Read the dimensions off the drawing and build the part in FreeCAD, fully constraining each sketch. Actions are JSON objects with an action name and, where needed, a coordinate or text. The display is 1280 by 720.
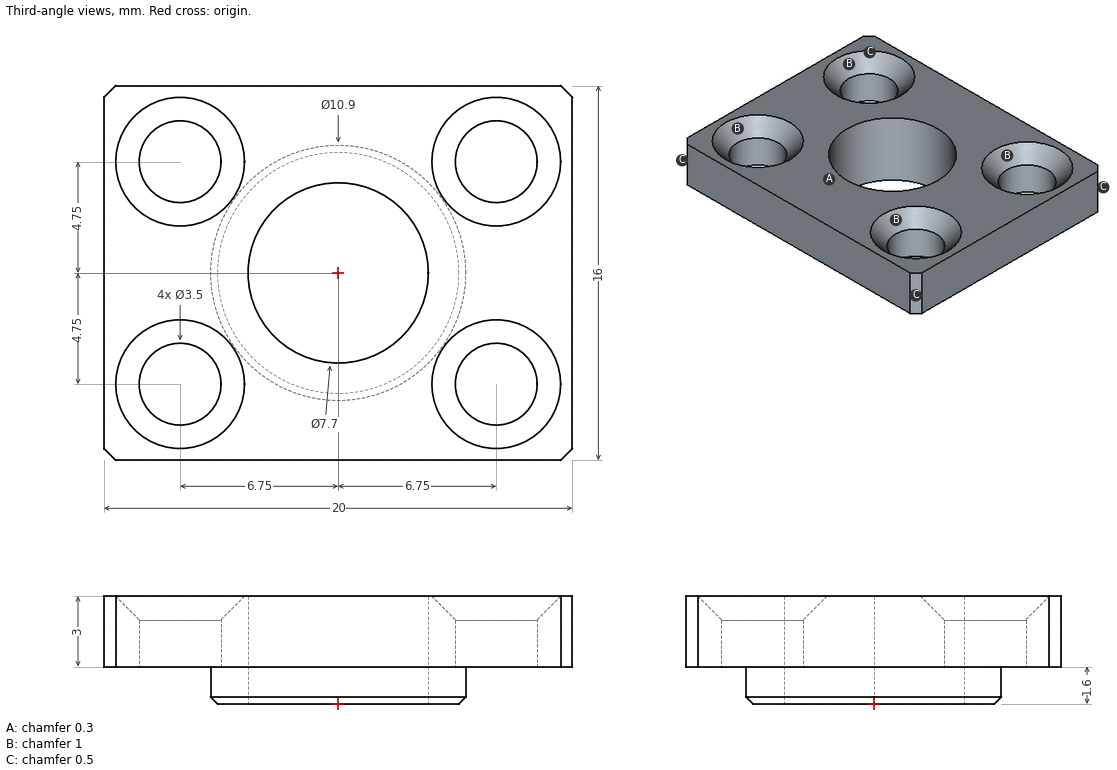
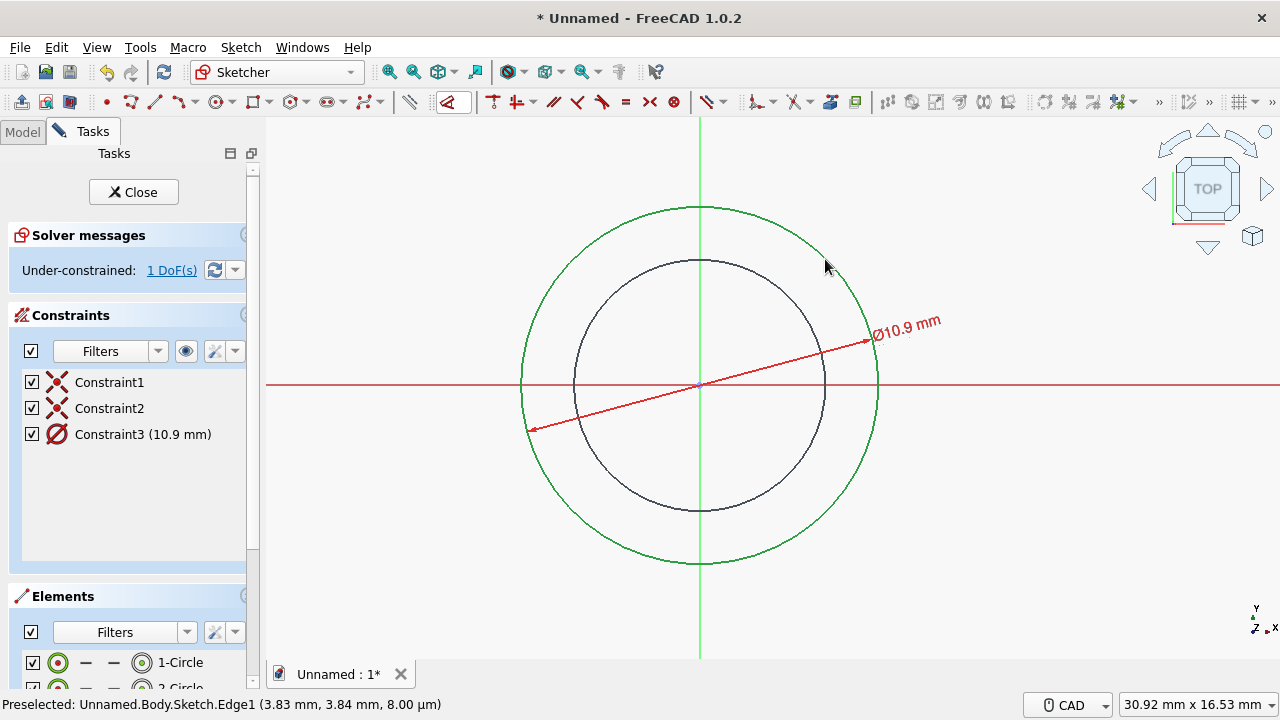
{"action": "left_click", "coordinate": [788, 296]}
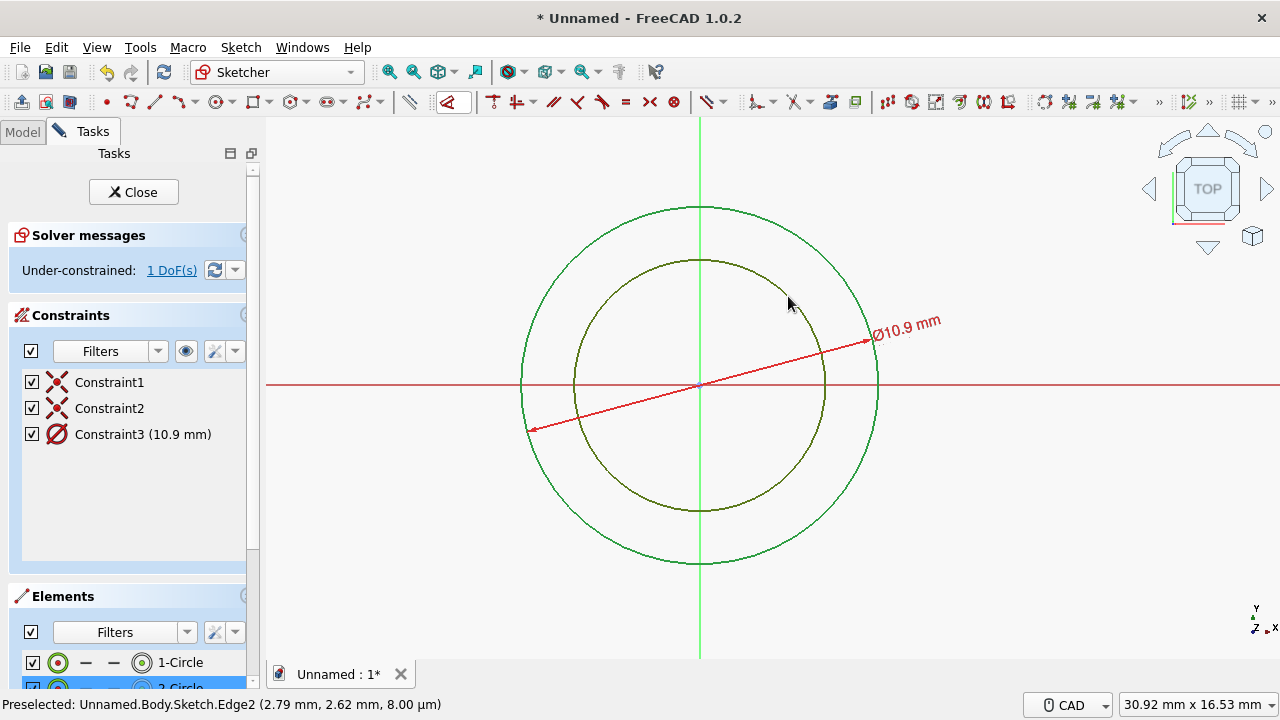
{"action": "key", "text": "k o"}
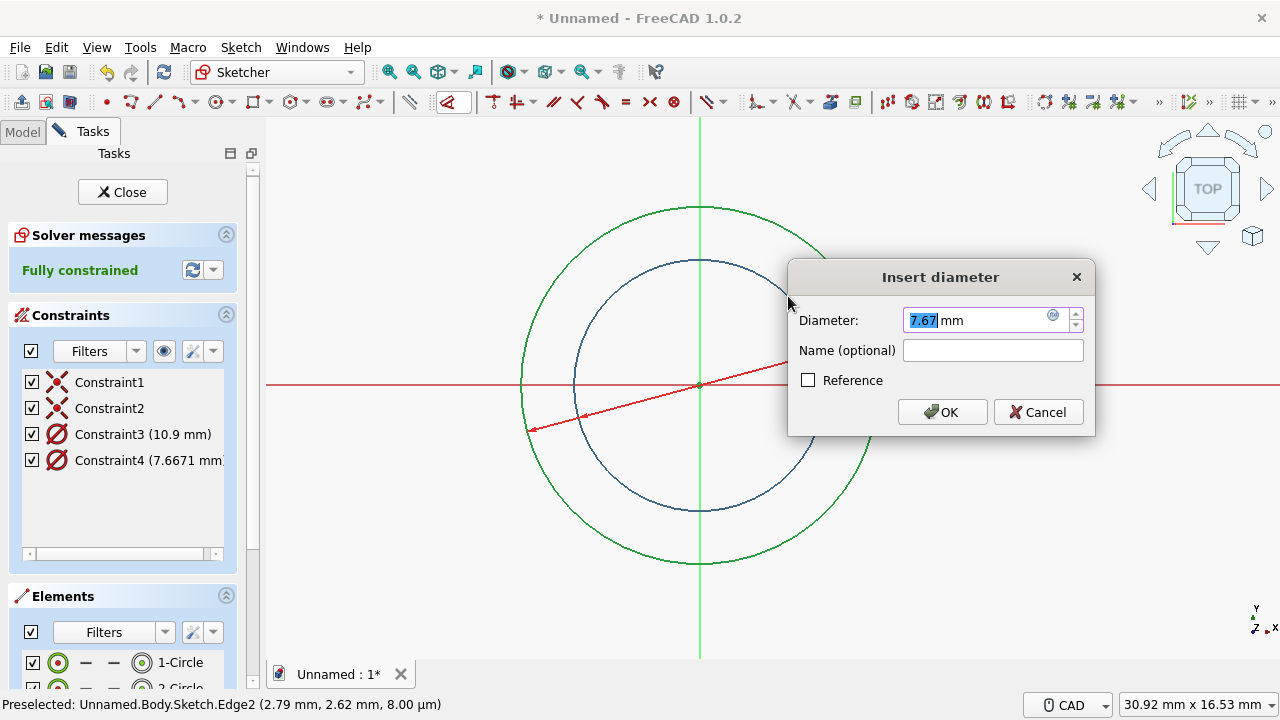
{"action": "type", "text": "7.7"}
{"action": "key", "text": "Return"}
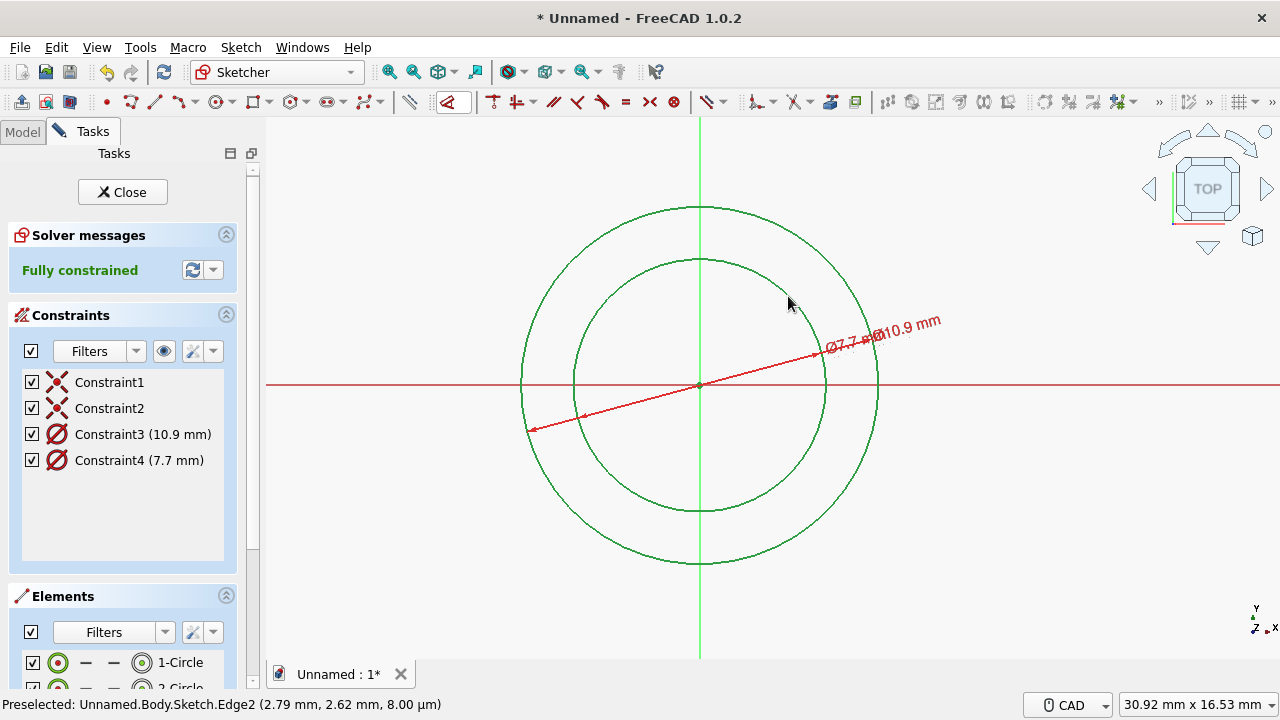
{"action": "left_click", "coordinate": [123, 192]}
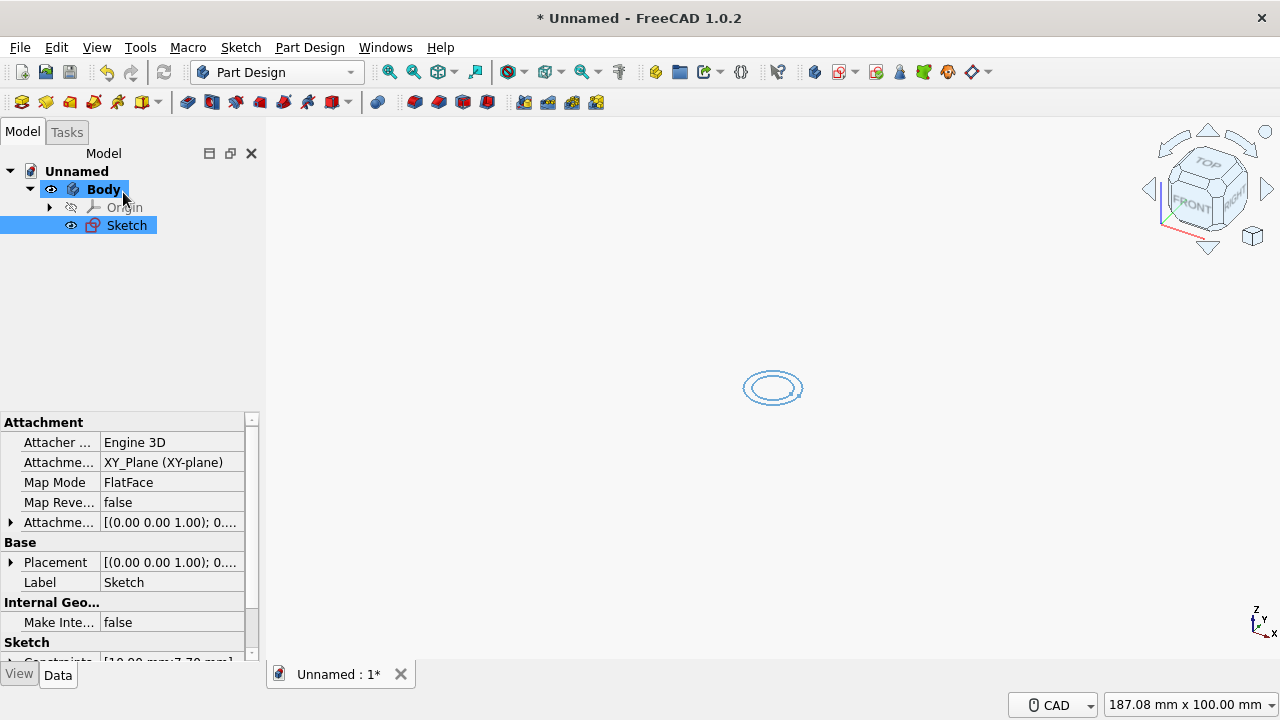
{"action": "left_click", "coordinate": [22, 102]}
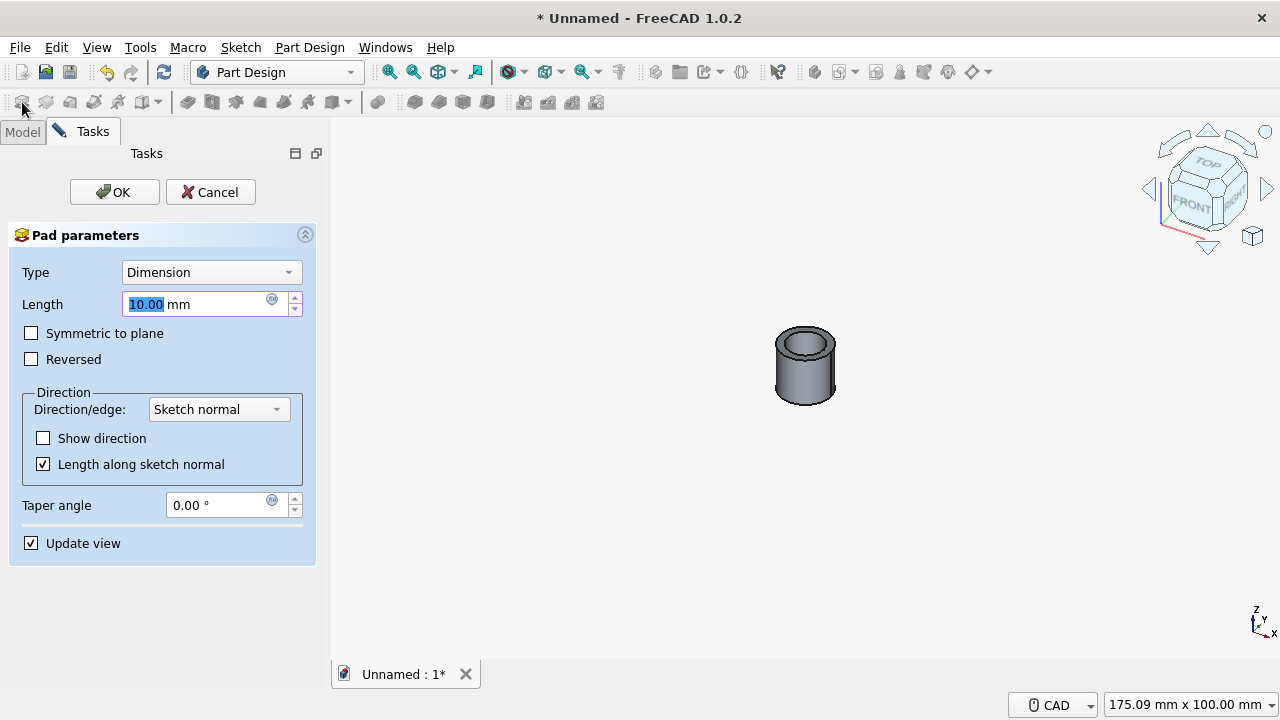
{"action": "type", "text": "1.6"}
{"action": "key", "text": "Tab"}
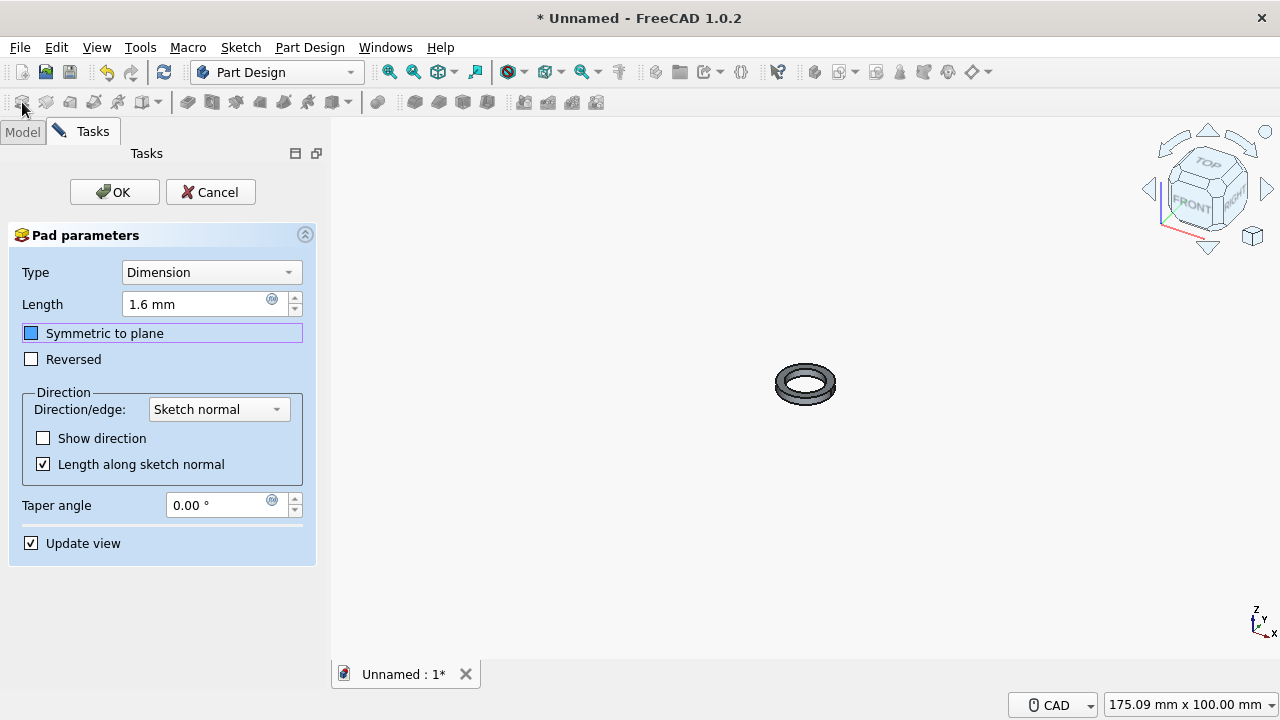
{"action": "left_click", "coordinate": [115, 192]}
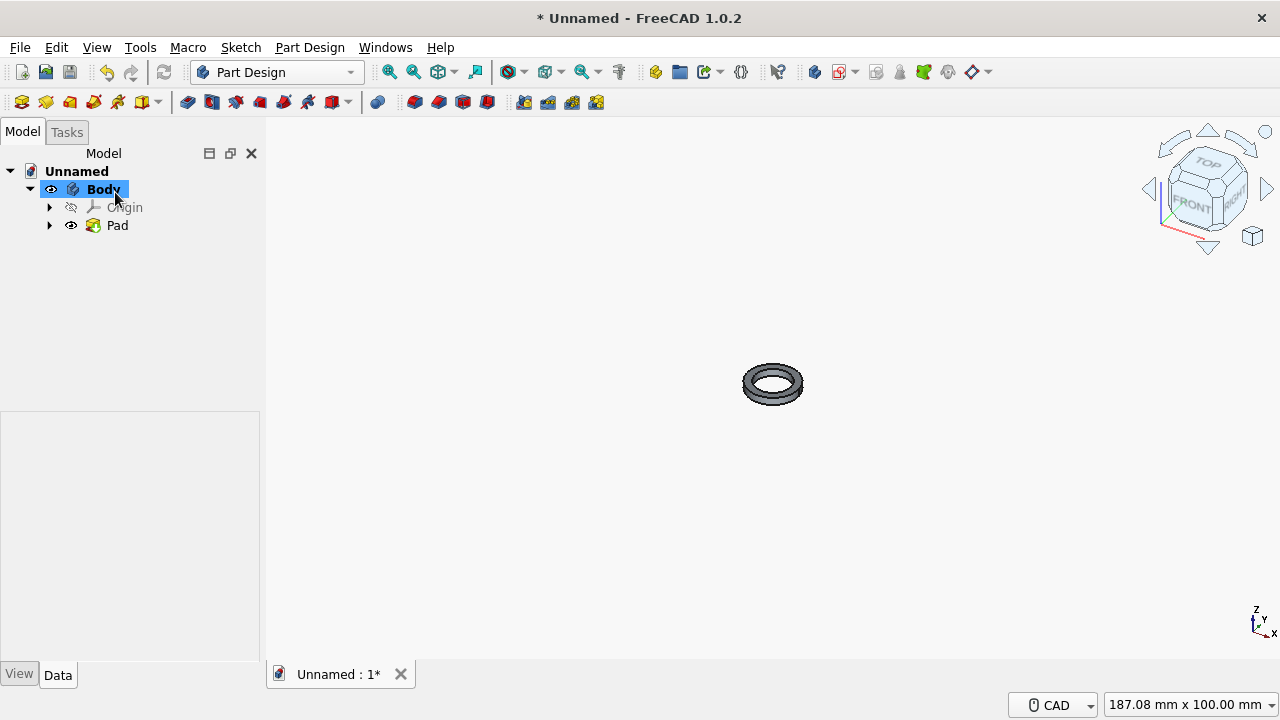
{"action": "key", "text": "v f"}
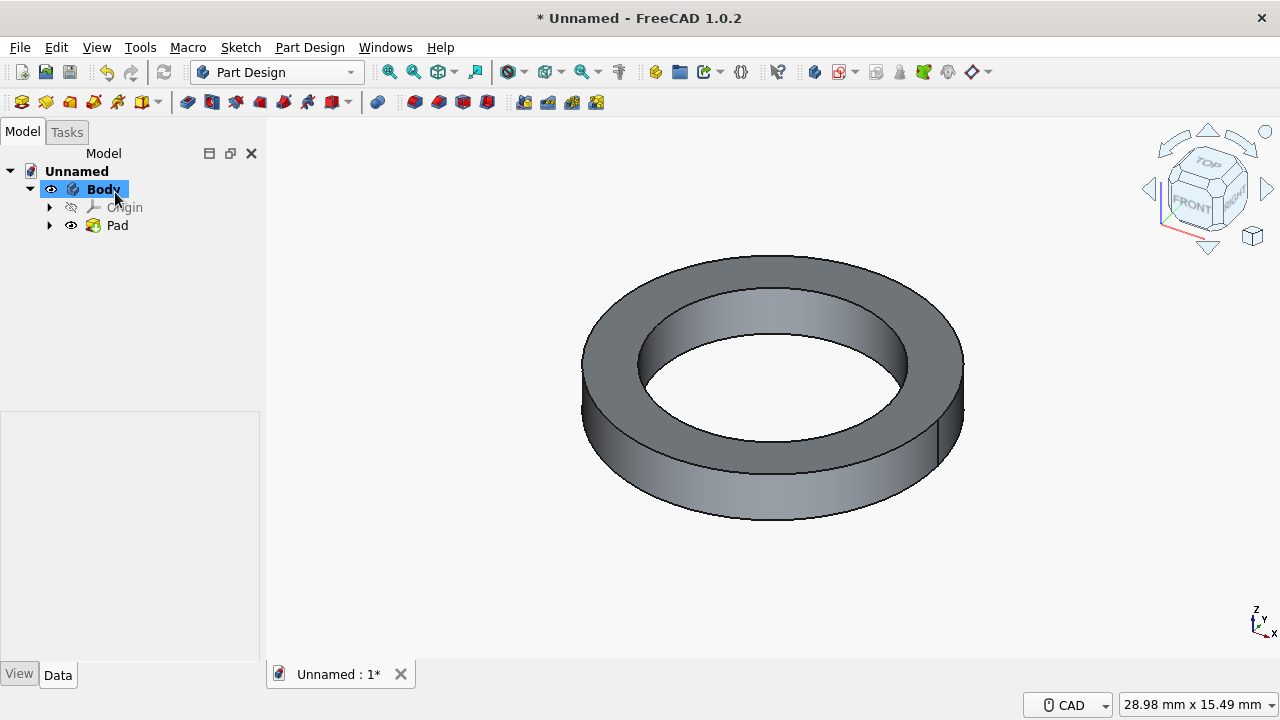
{"action": "left_click", "coordinate": [914, 411]}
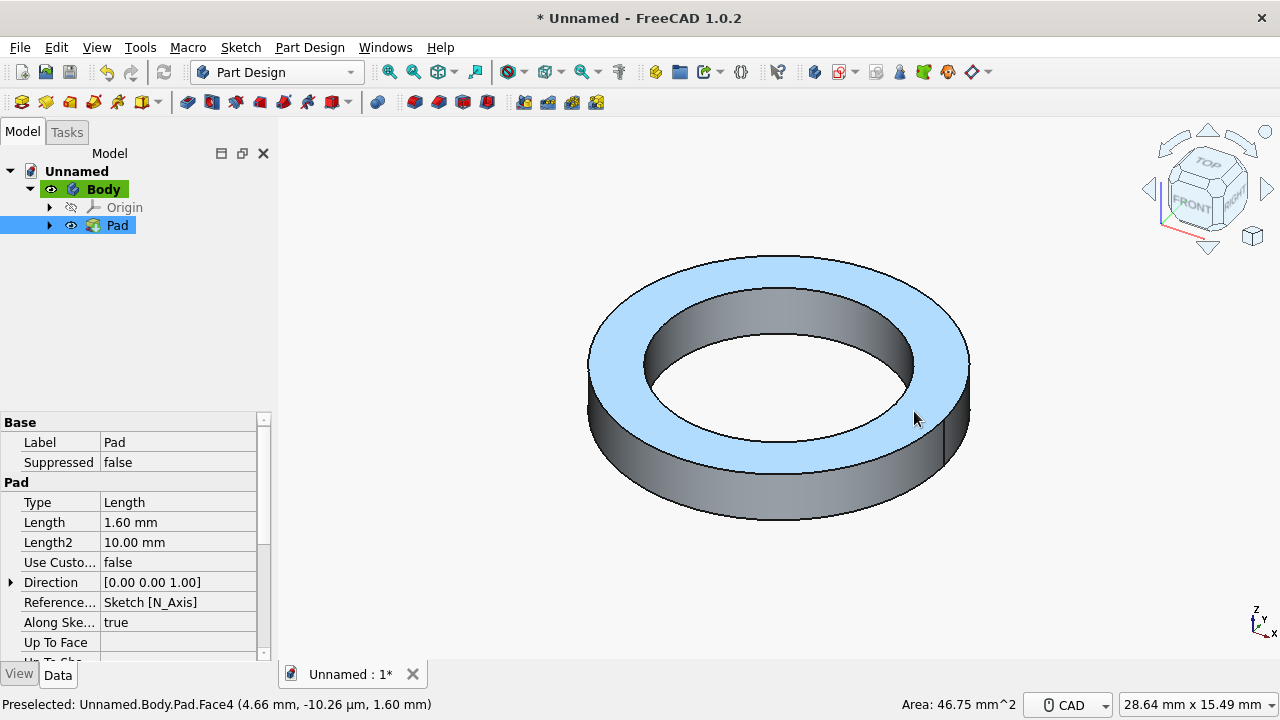
{"action": "left_click", "coordinate": [840, 72]}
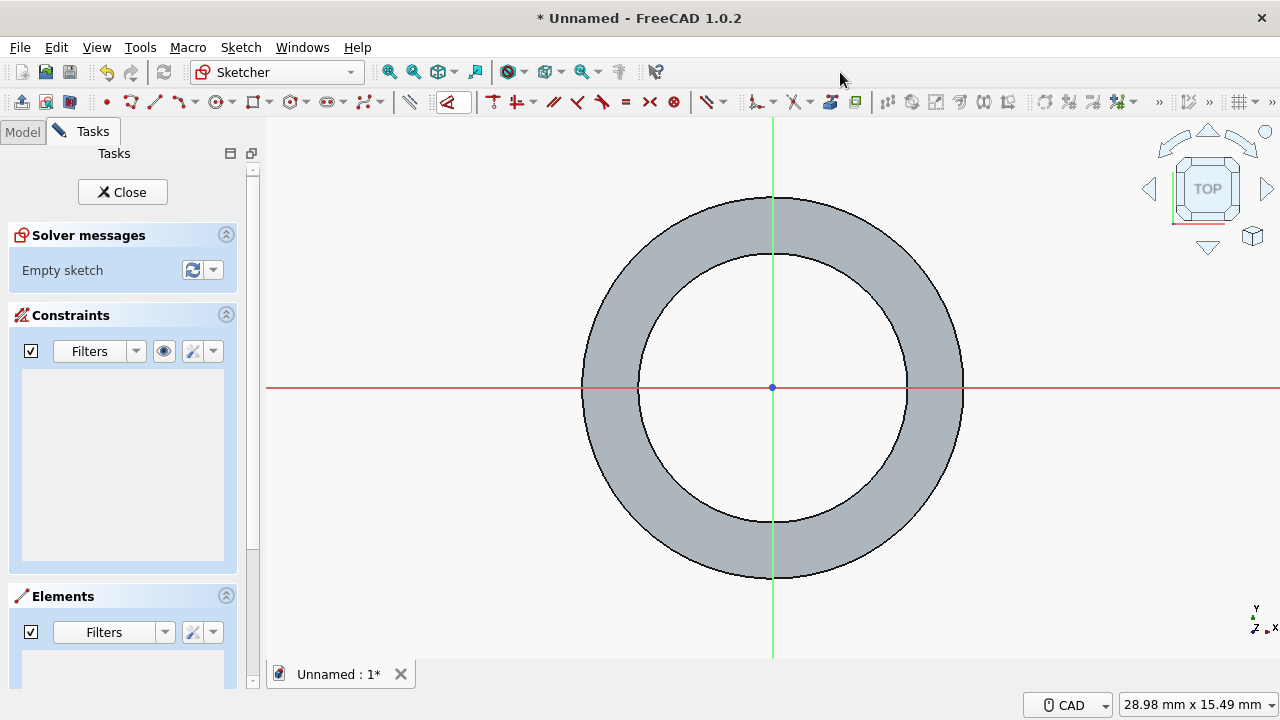
{"action": "scroll", "coordinate": [565, 388], "scroll_direction": "down", "scroll_amount": 2}